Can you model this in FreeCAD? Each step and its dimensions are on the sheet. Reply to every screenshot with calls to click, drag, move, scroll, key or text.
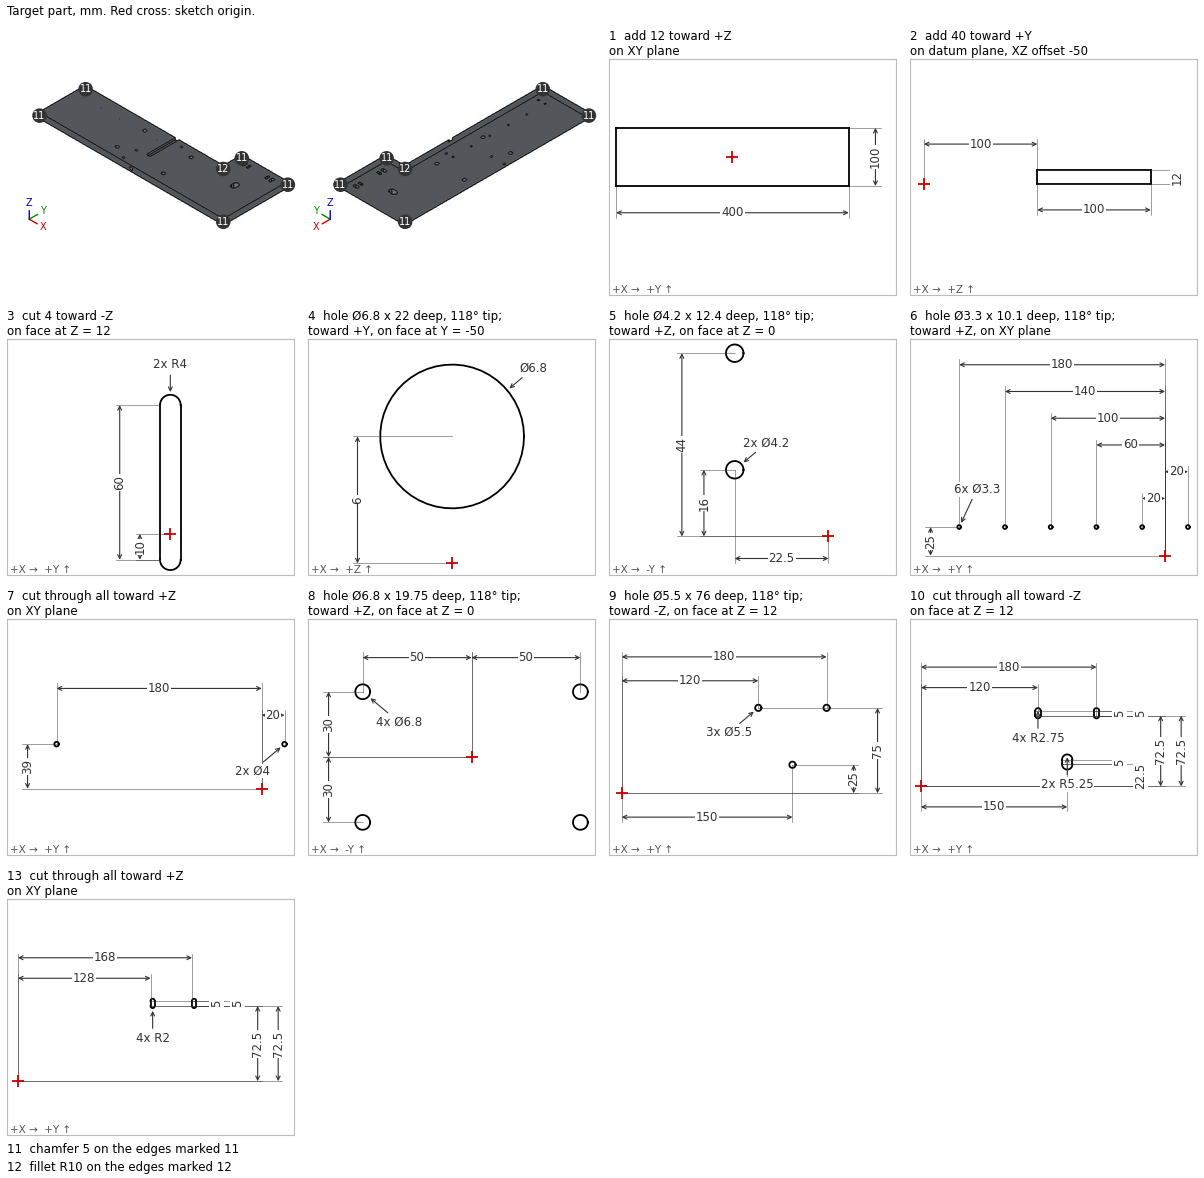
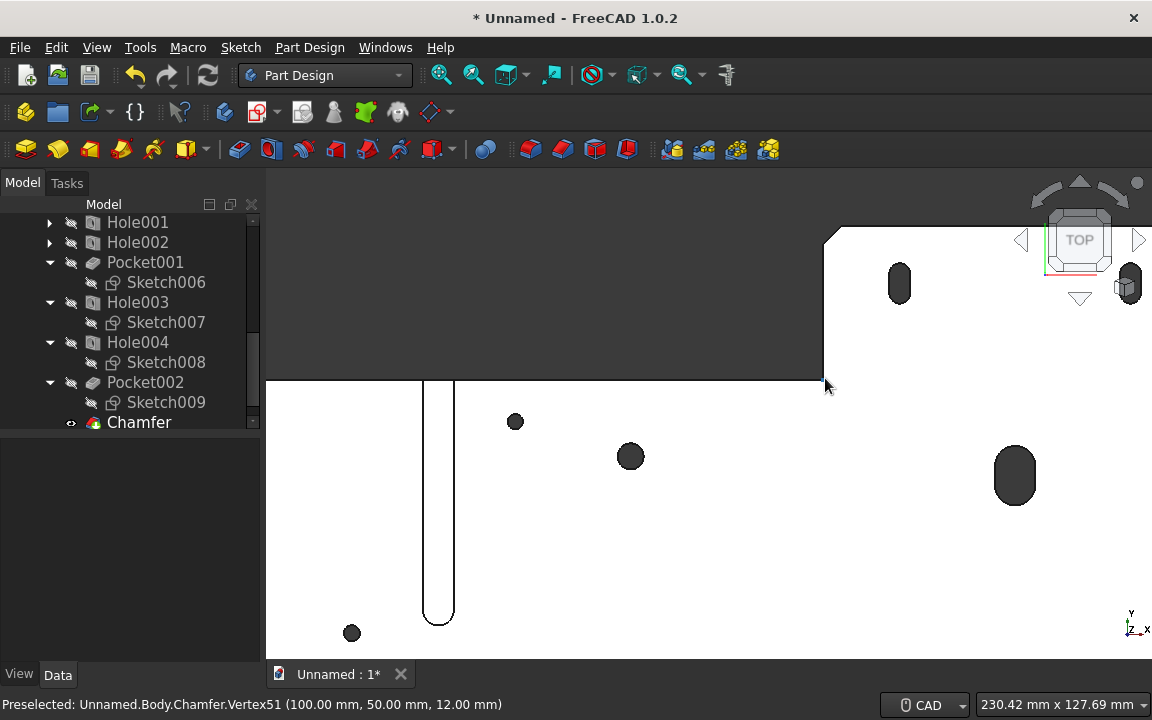
click(442, 76)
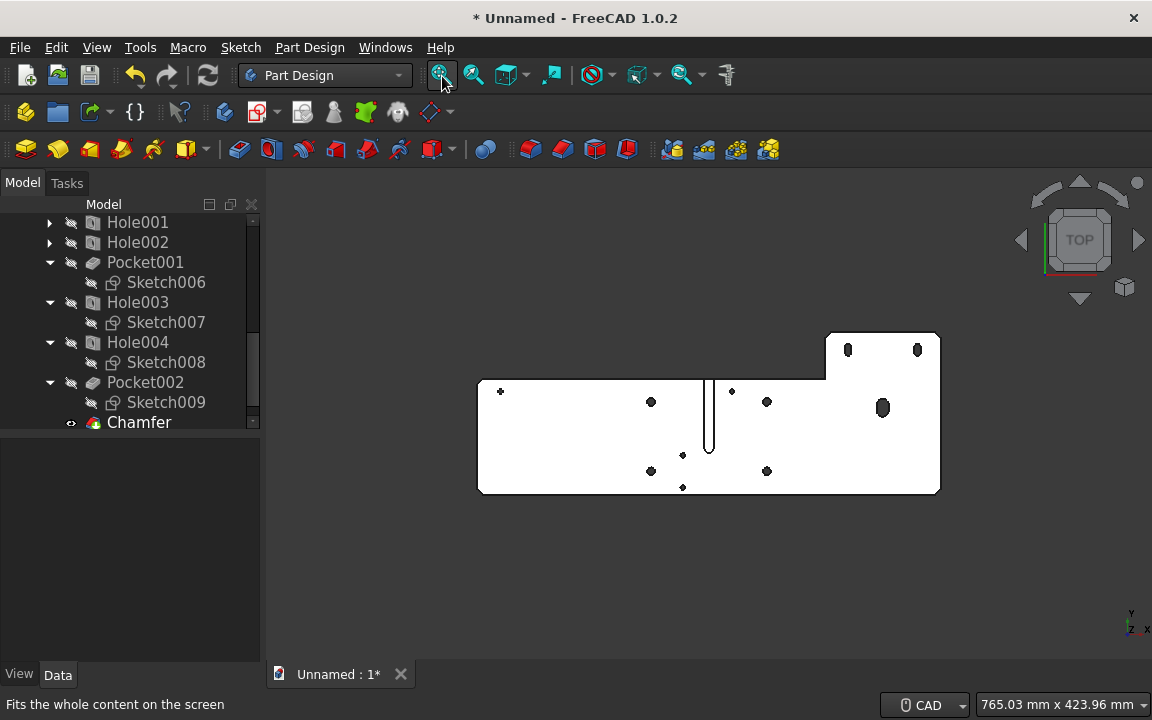
key(1)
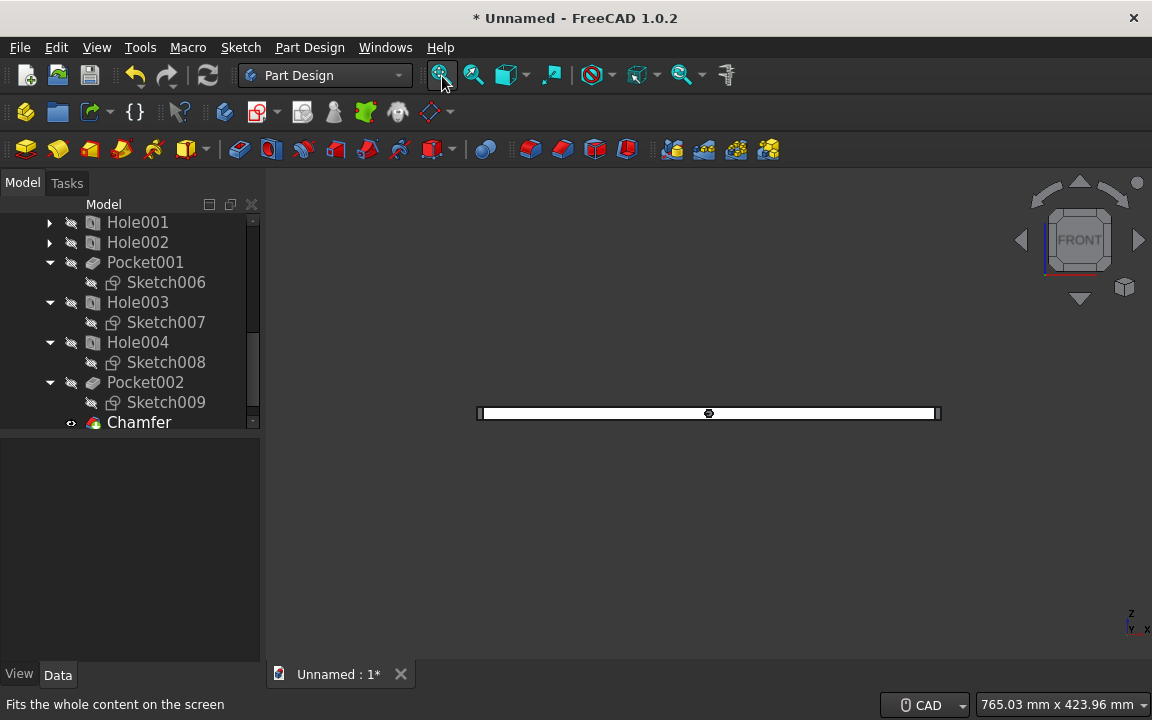
scroll(825, 412, up, 6)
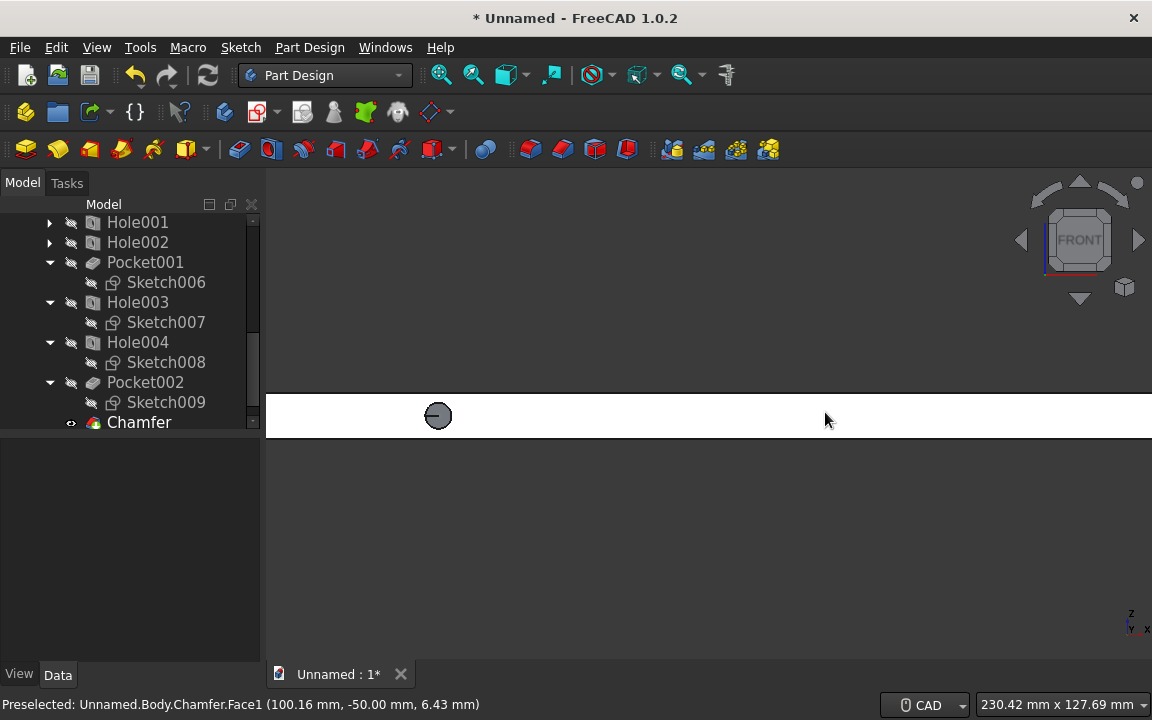
click(442, 76)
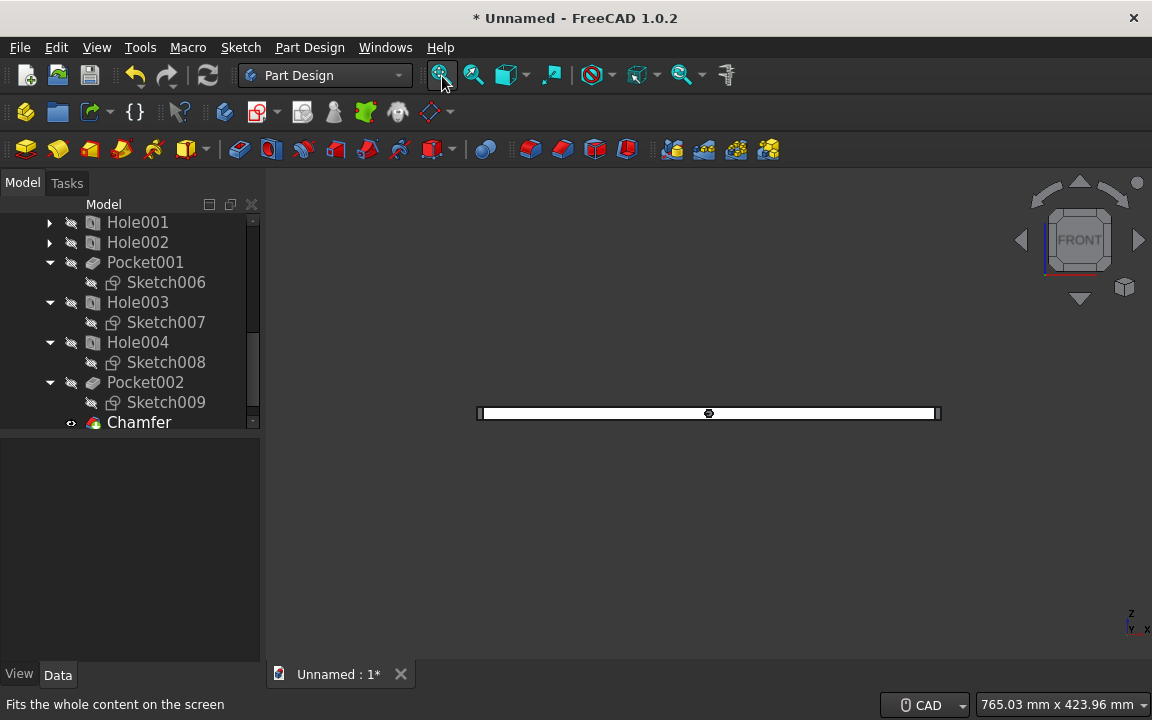
key(3)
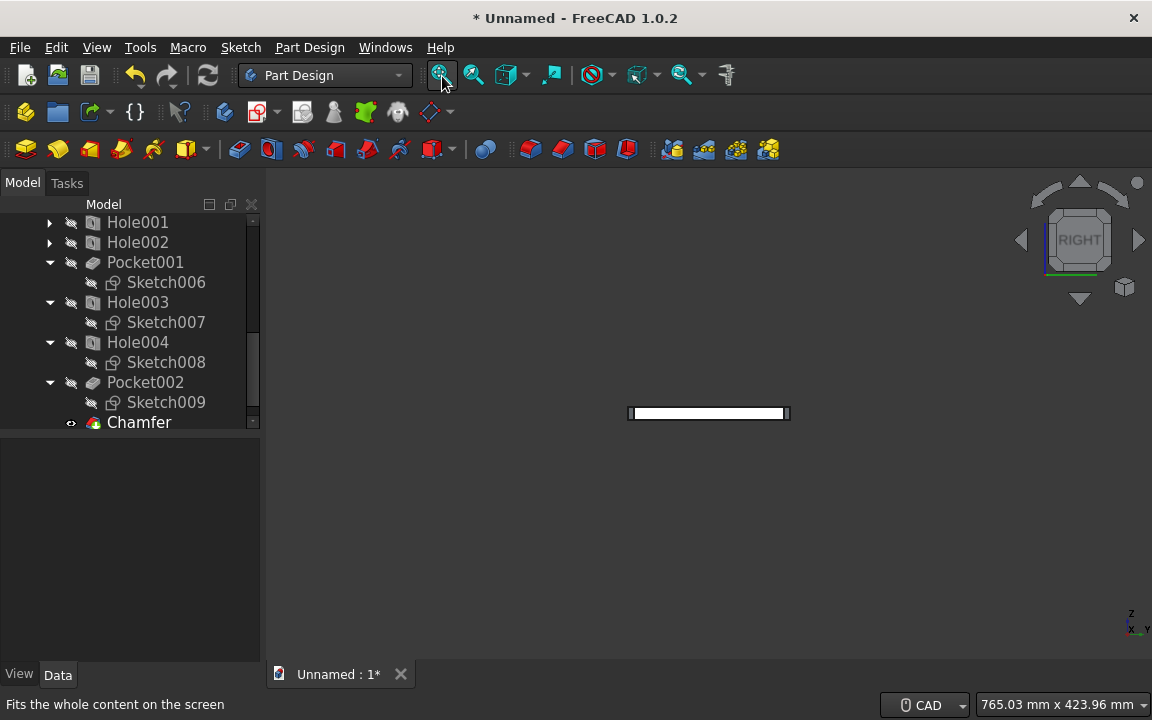
click(442, 76)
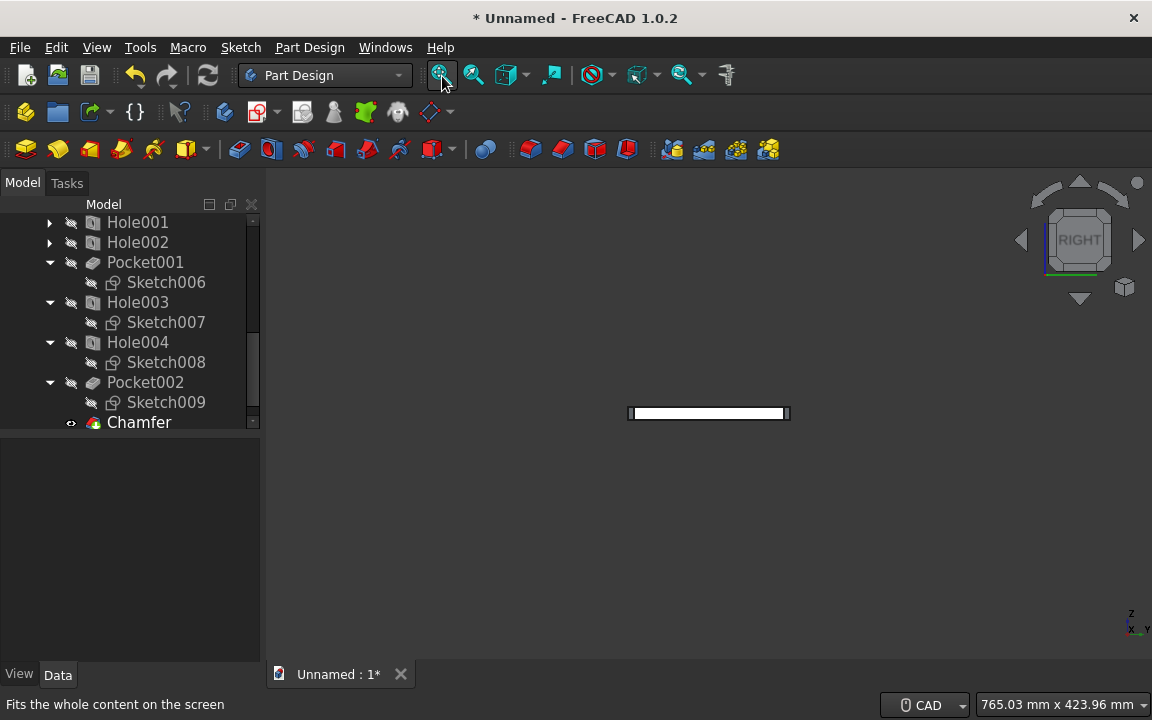
scroll(744, 412, up, 6)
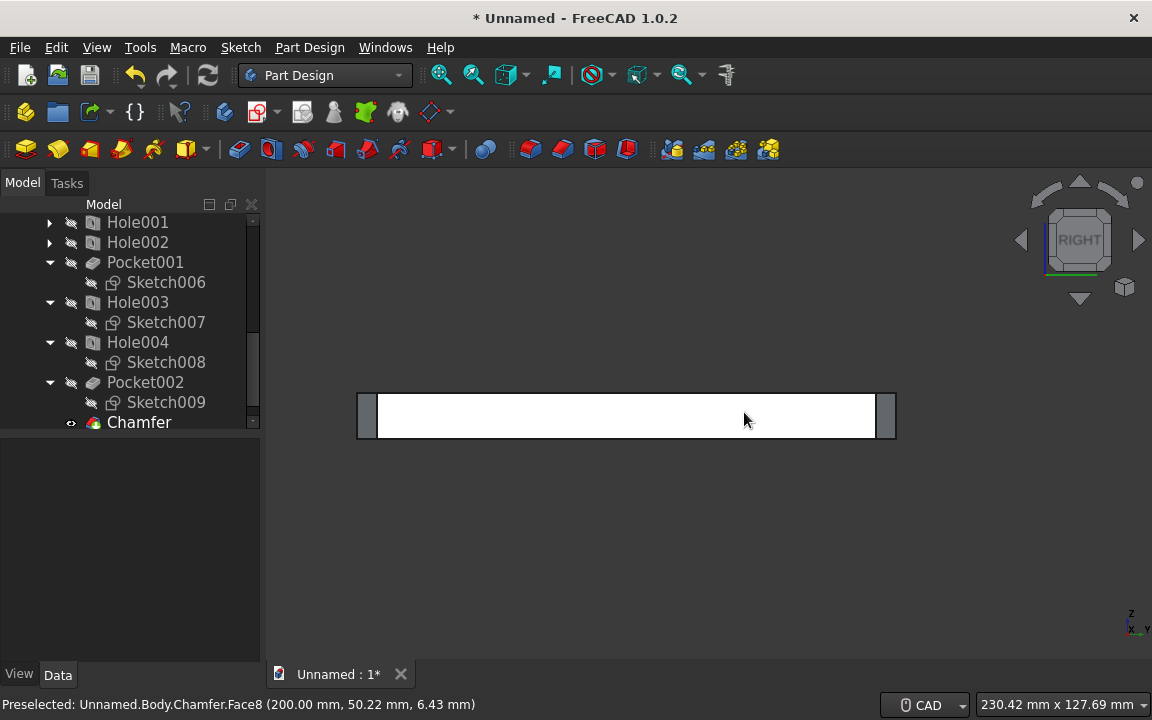
click(442, 76)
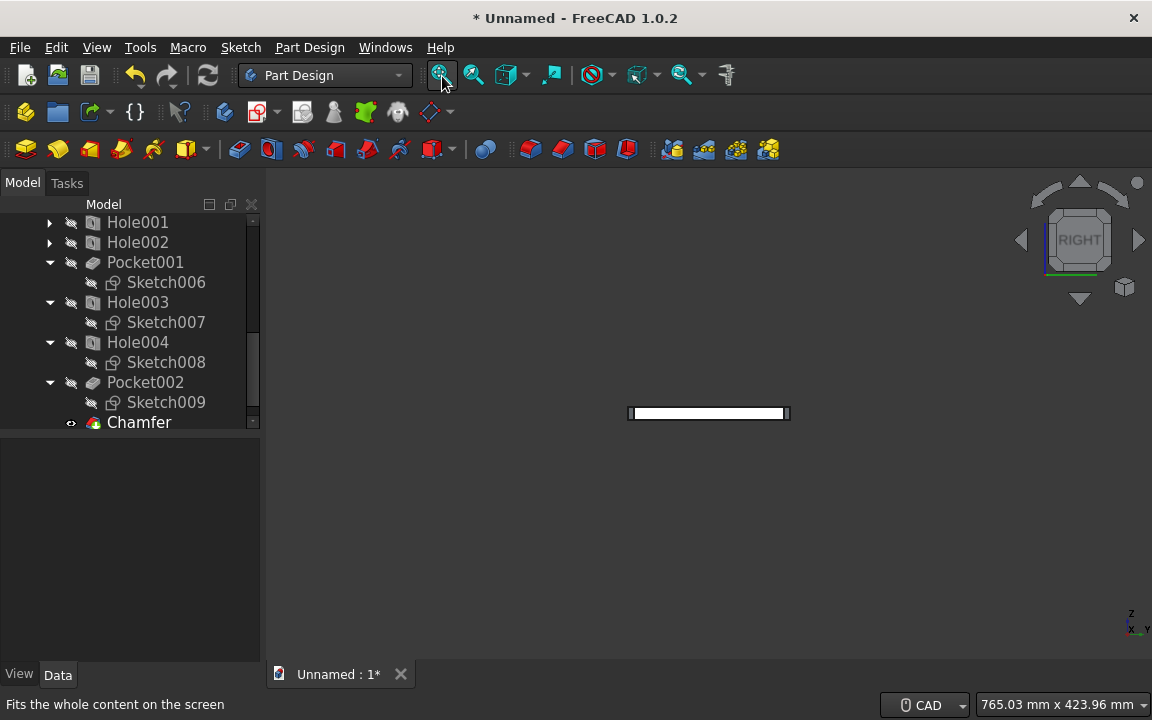
key(5)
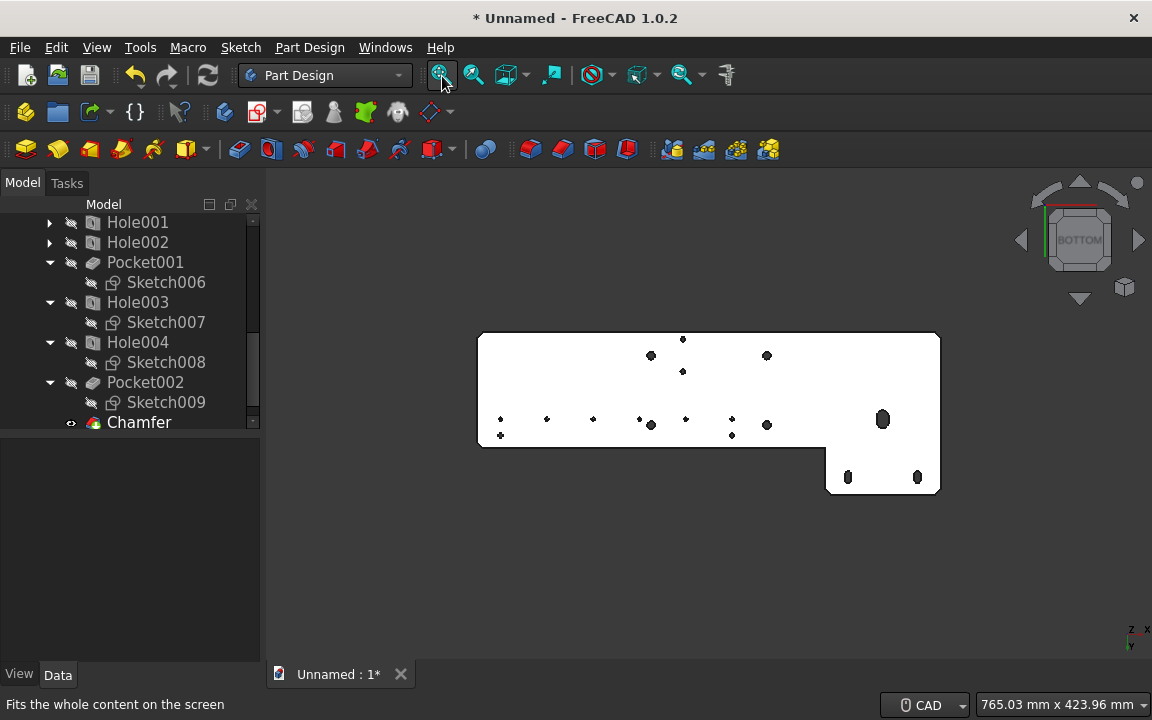
scroll(825, 447, up, 6)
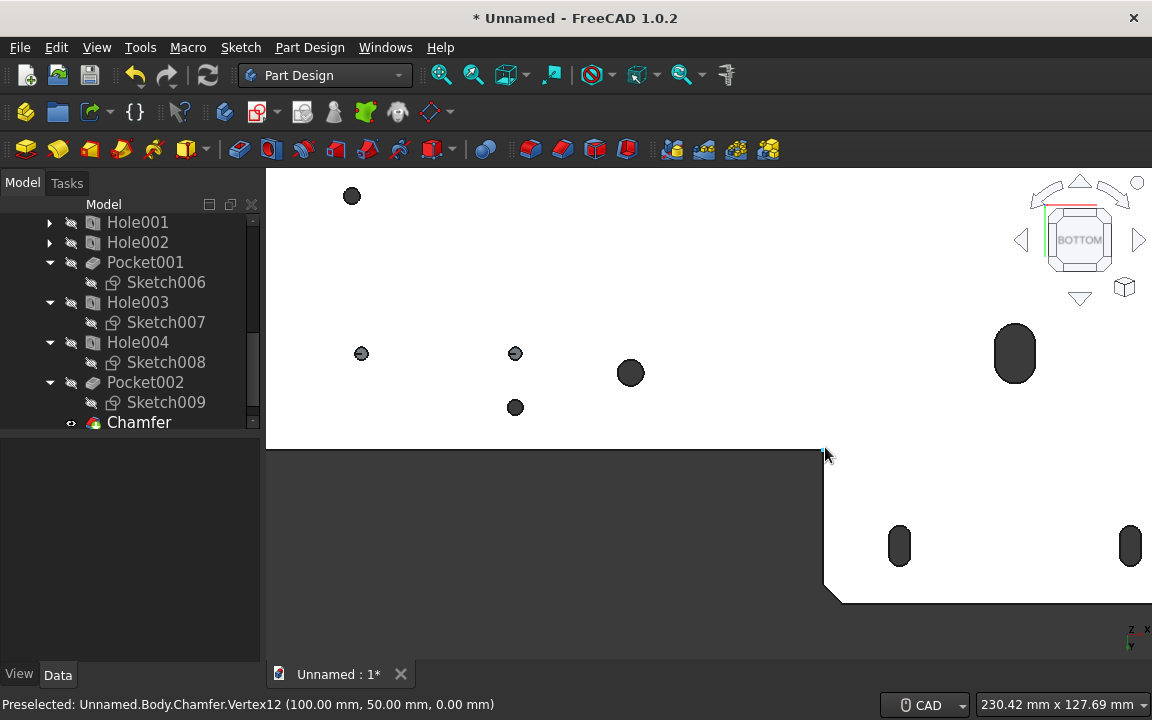
click(442, 76)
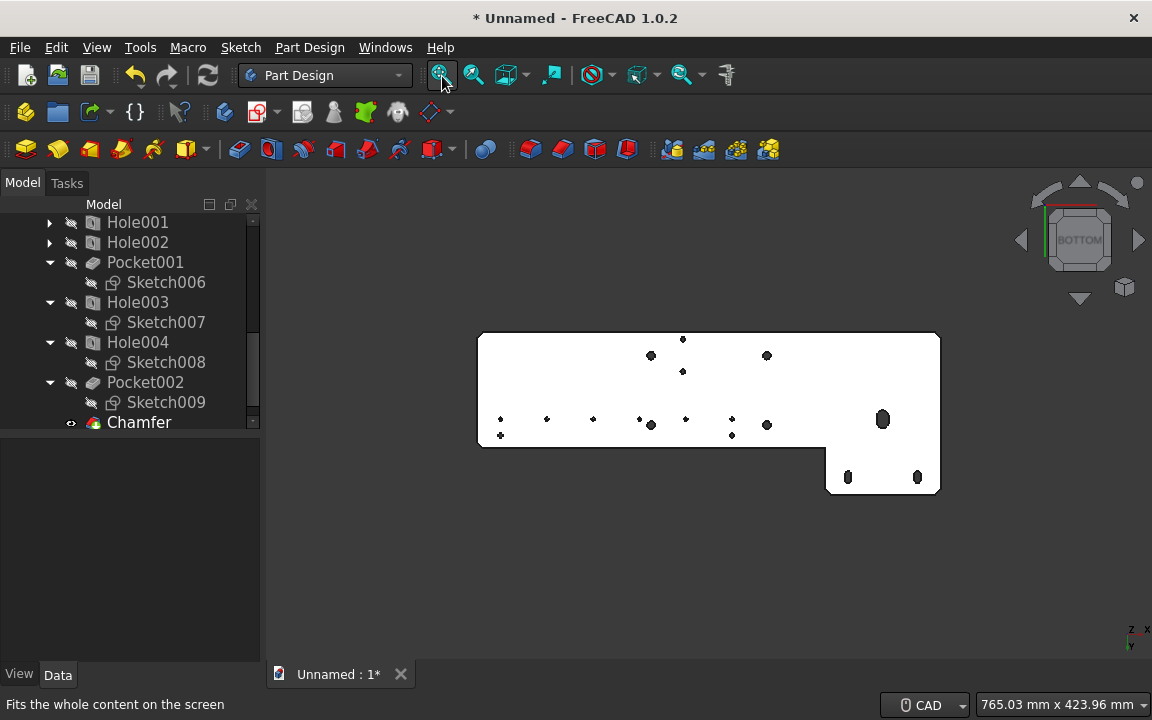
key(4)